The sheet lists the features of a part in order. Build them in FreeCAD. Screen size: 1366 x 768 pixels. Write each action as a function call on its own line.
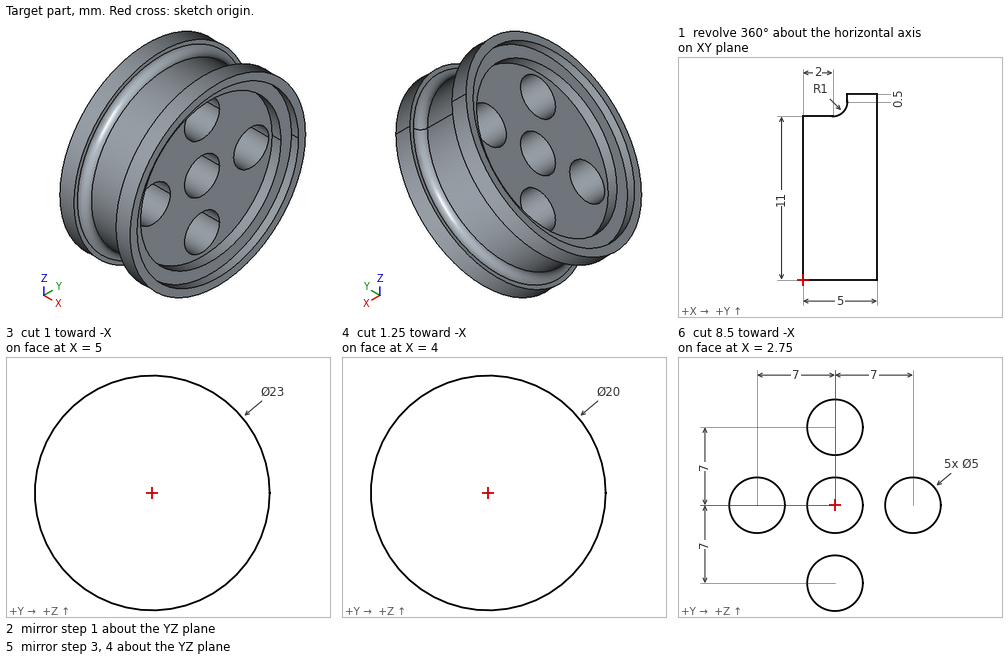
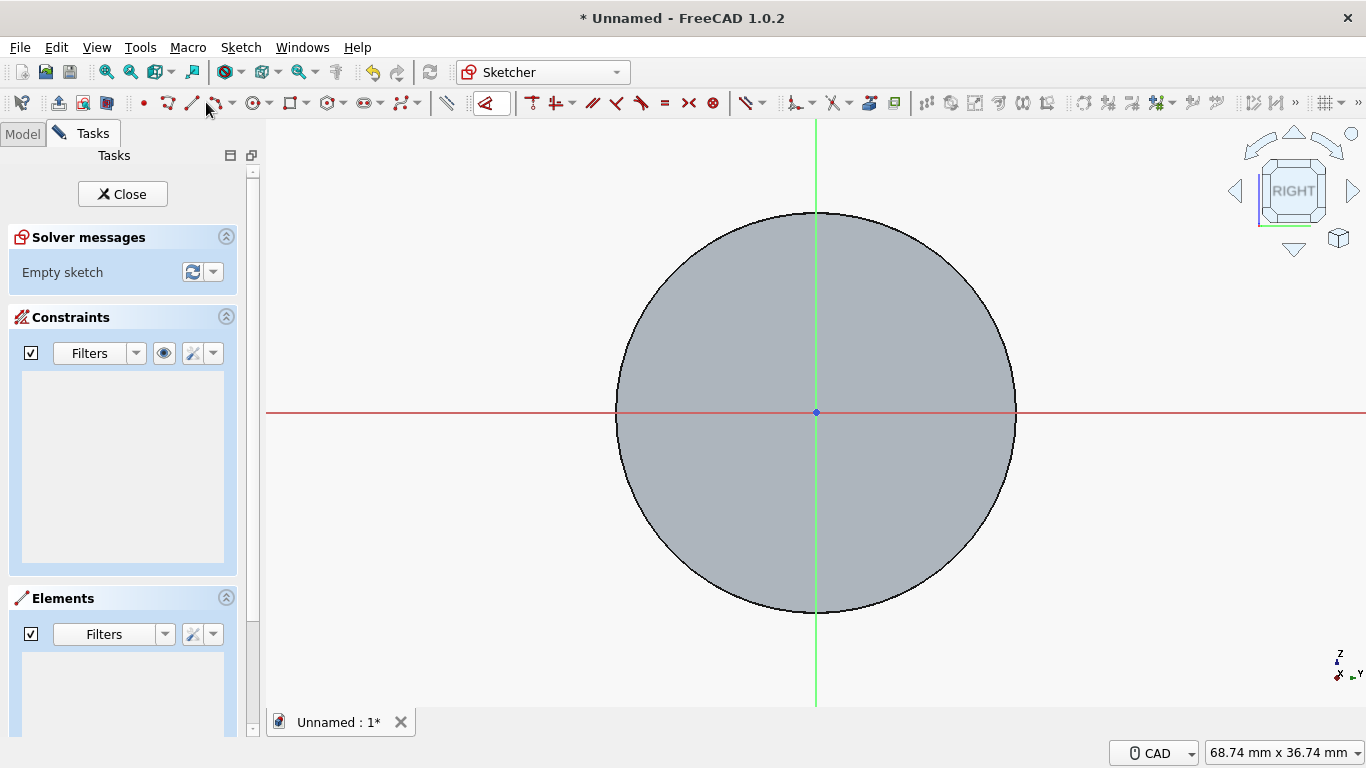
key(g)
key(c)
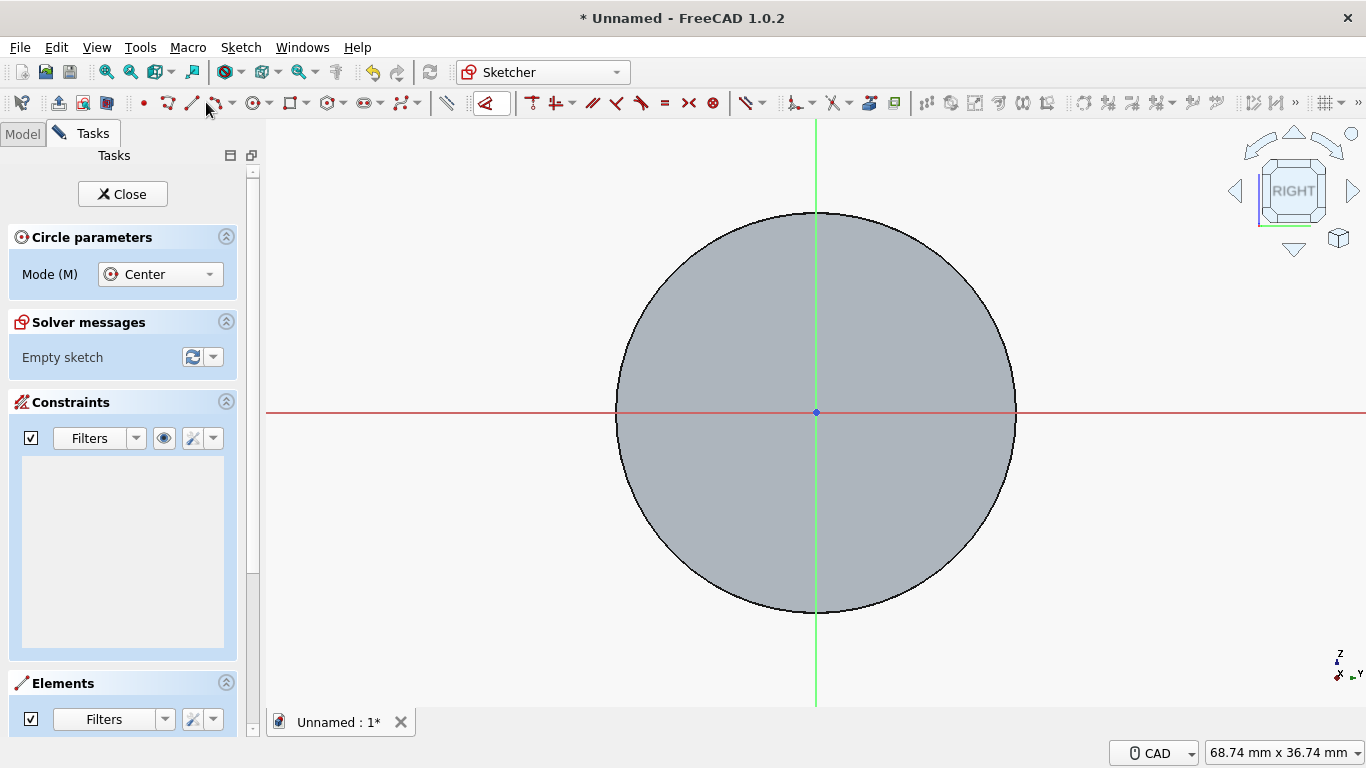
click(816, 413)
click(946, 283)
key(Escape)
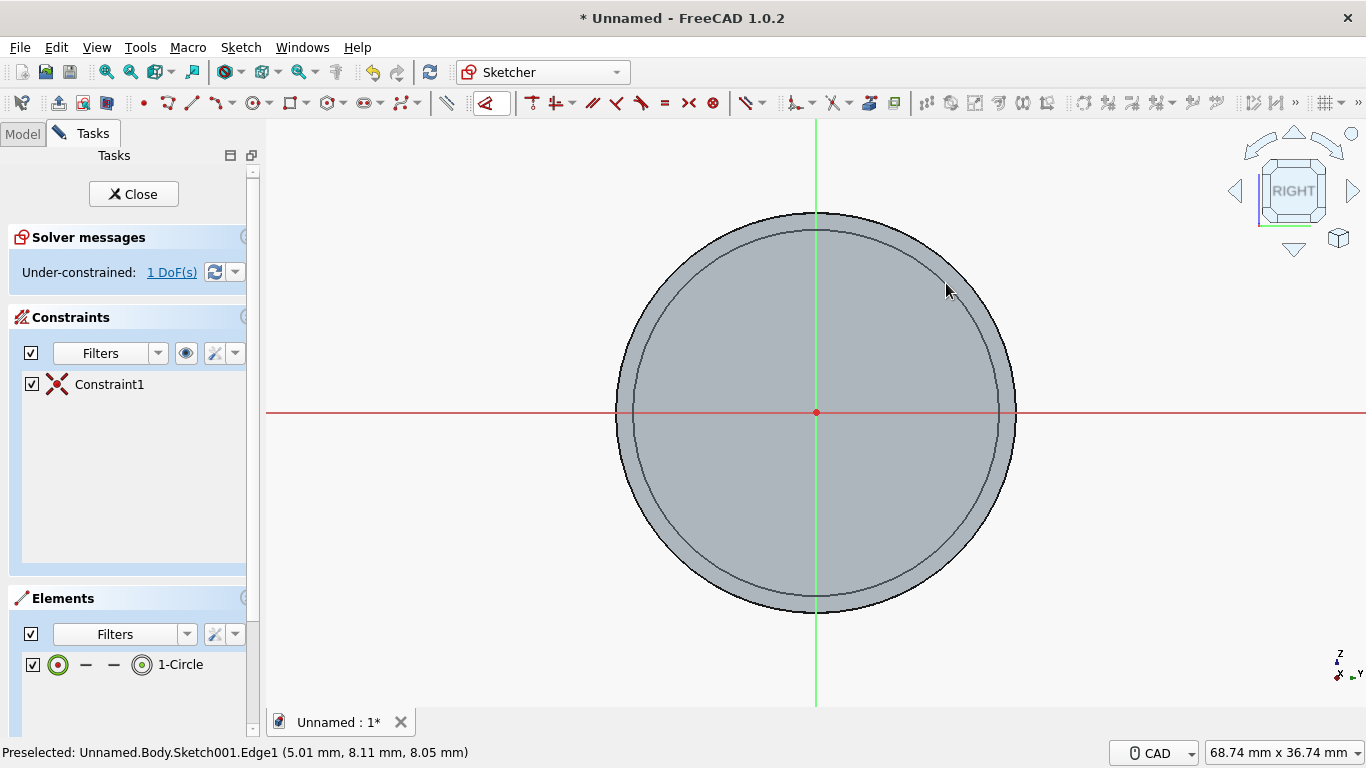
click(486, 104)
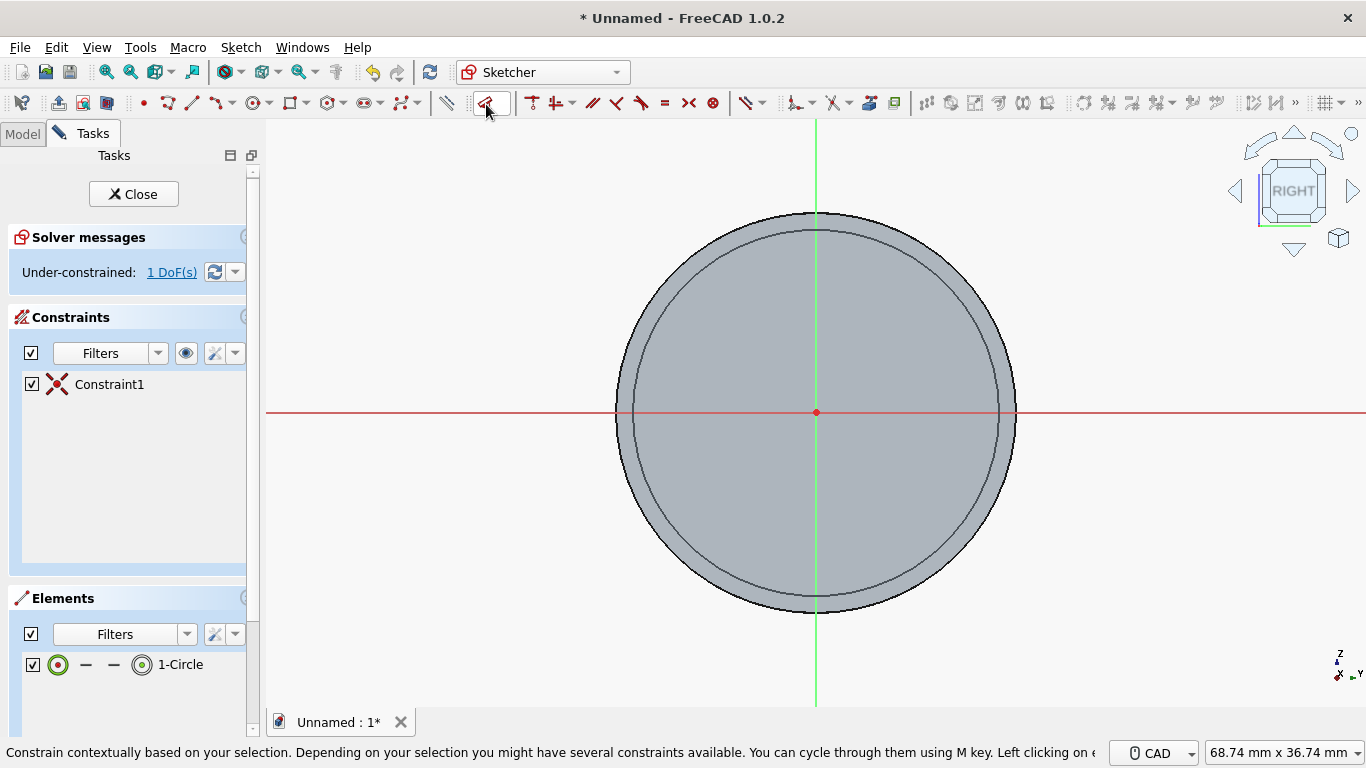
click(945, 283)
click(968, 260)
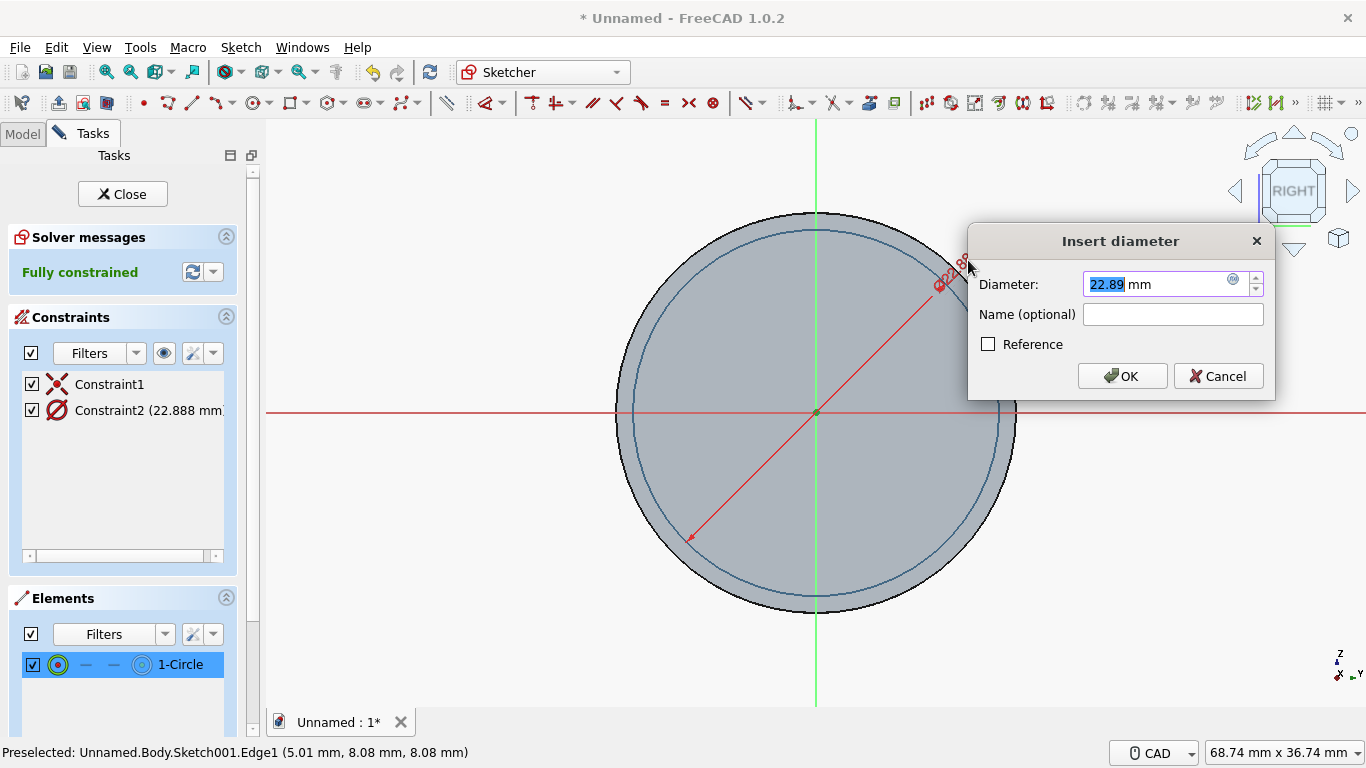
text(23)
key(Return)
key(Escape)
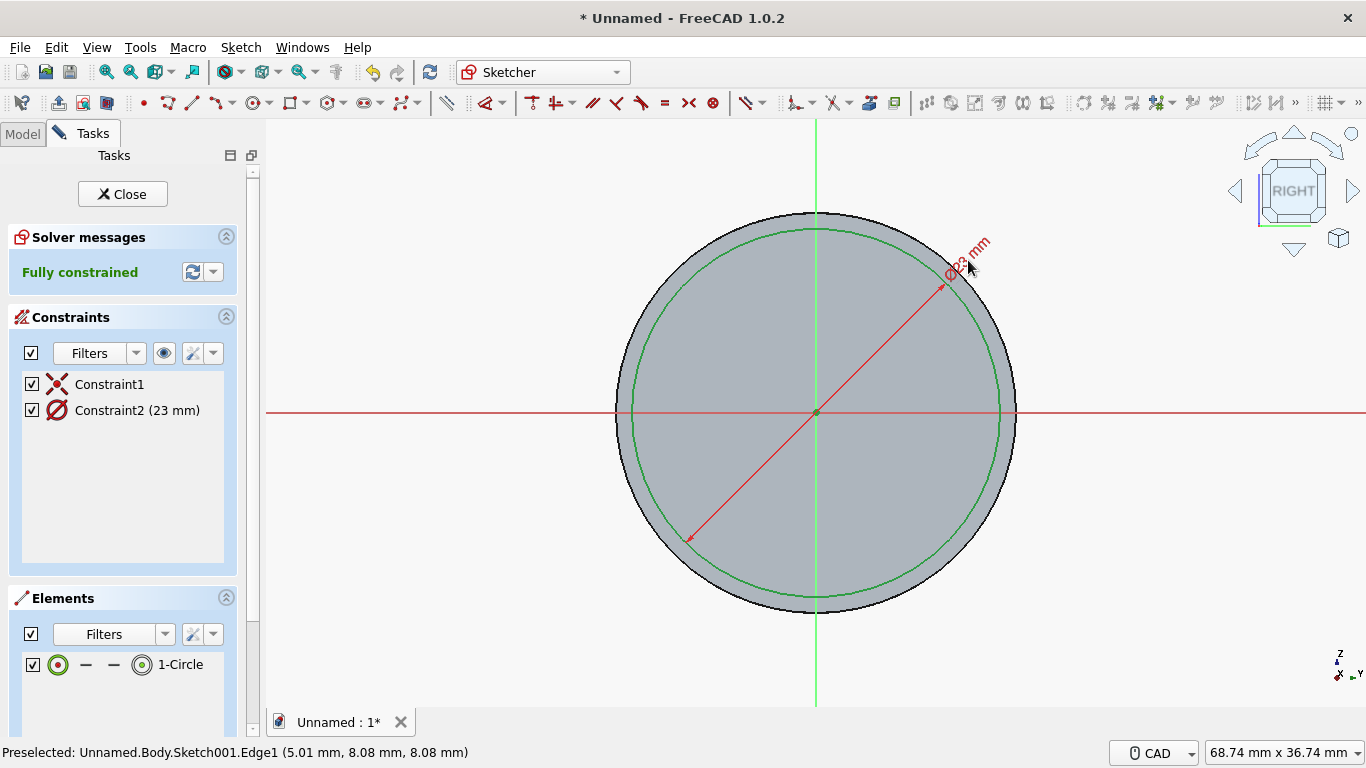
click(123, 194)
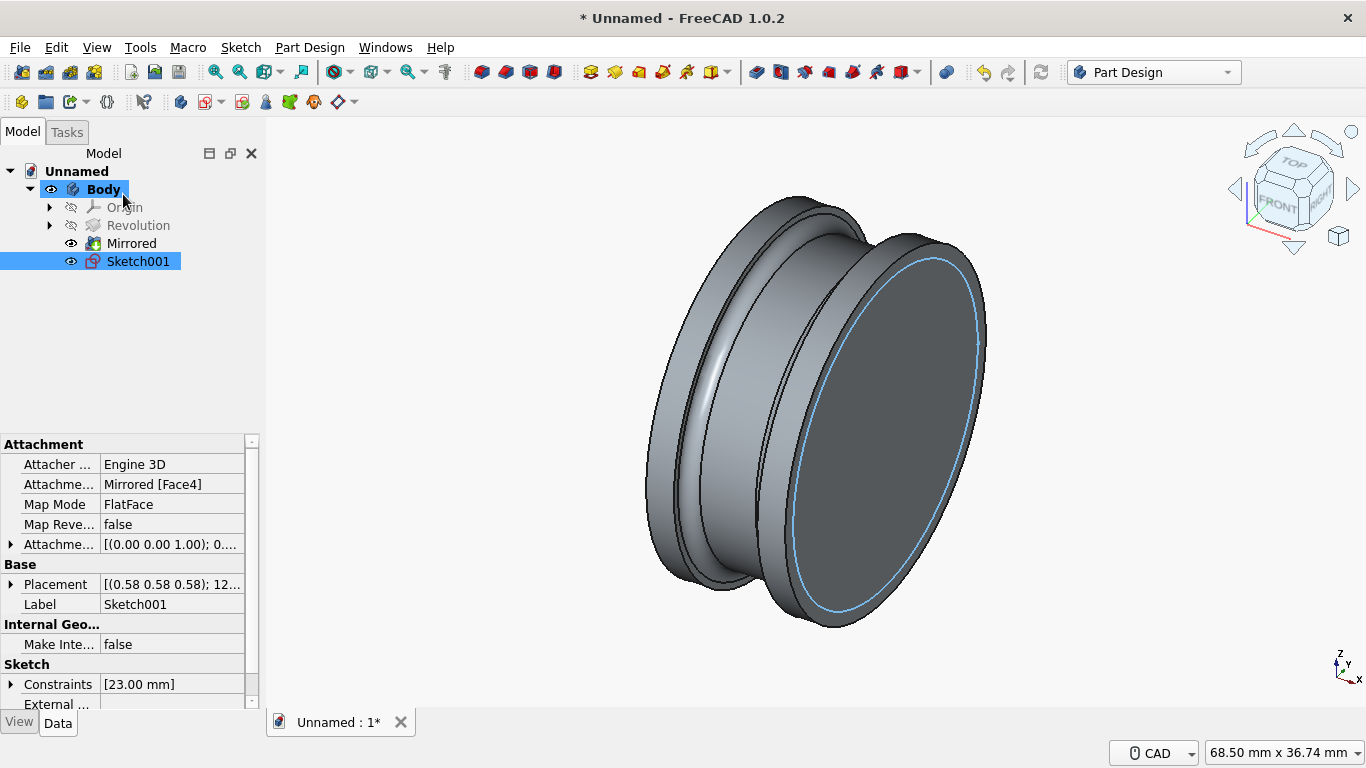
click(758, 72)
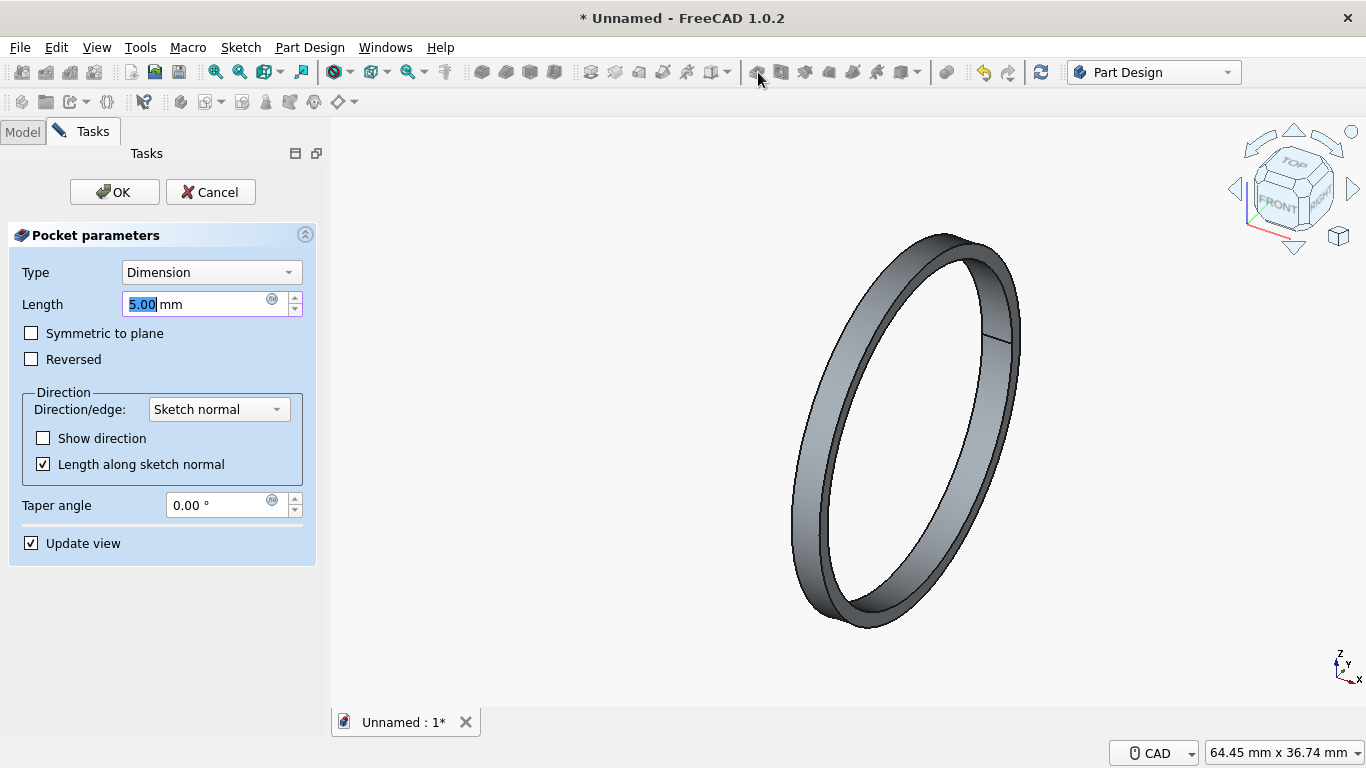
text(1)
key(Tab)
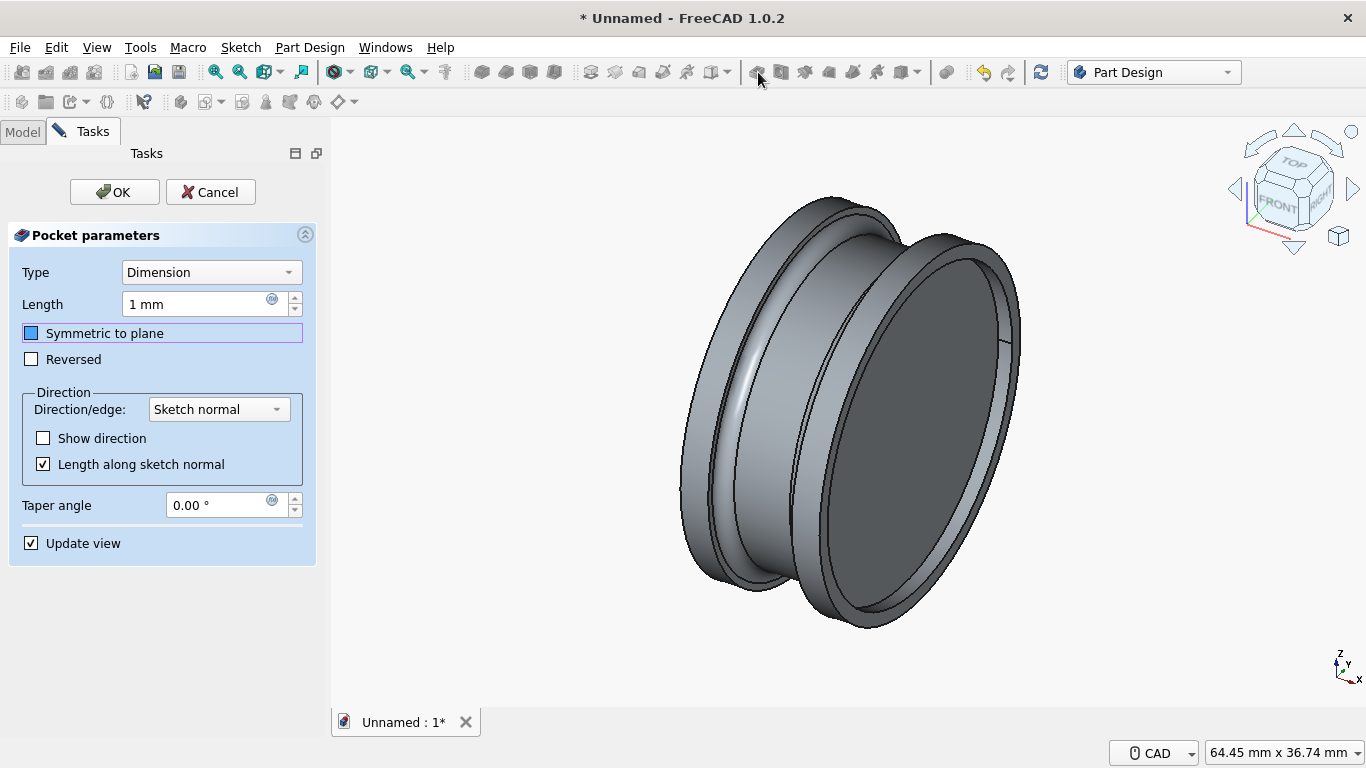
click(115, 192)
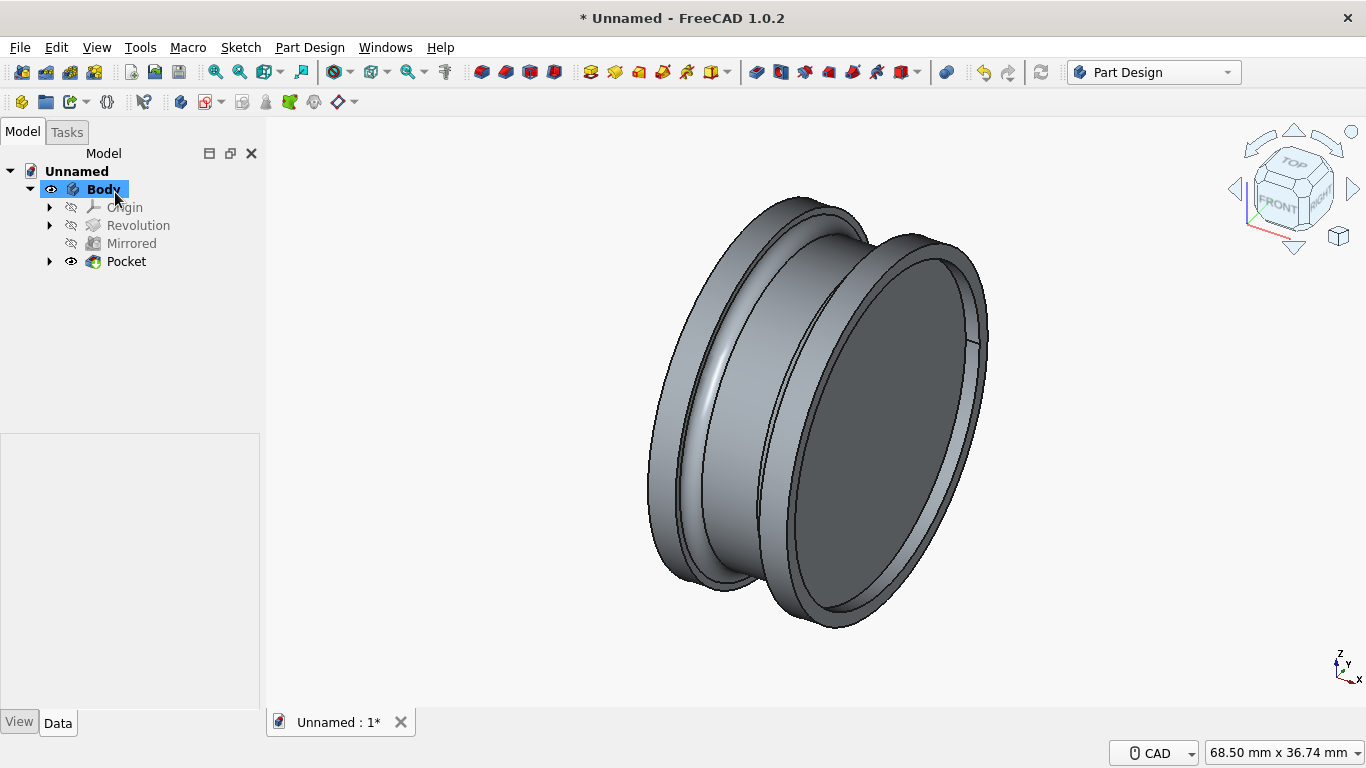
click(873, 430)